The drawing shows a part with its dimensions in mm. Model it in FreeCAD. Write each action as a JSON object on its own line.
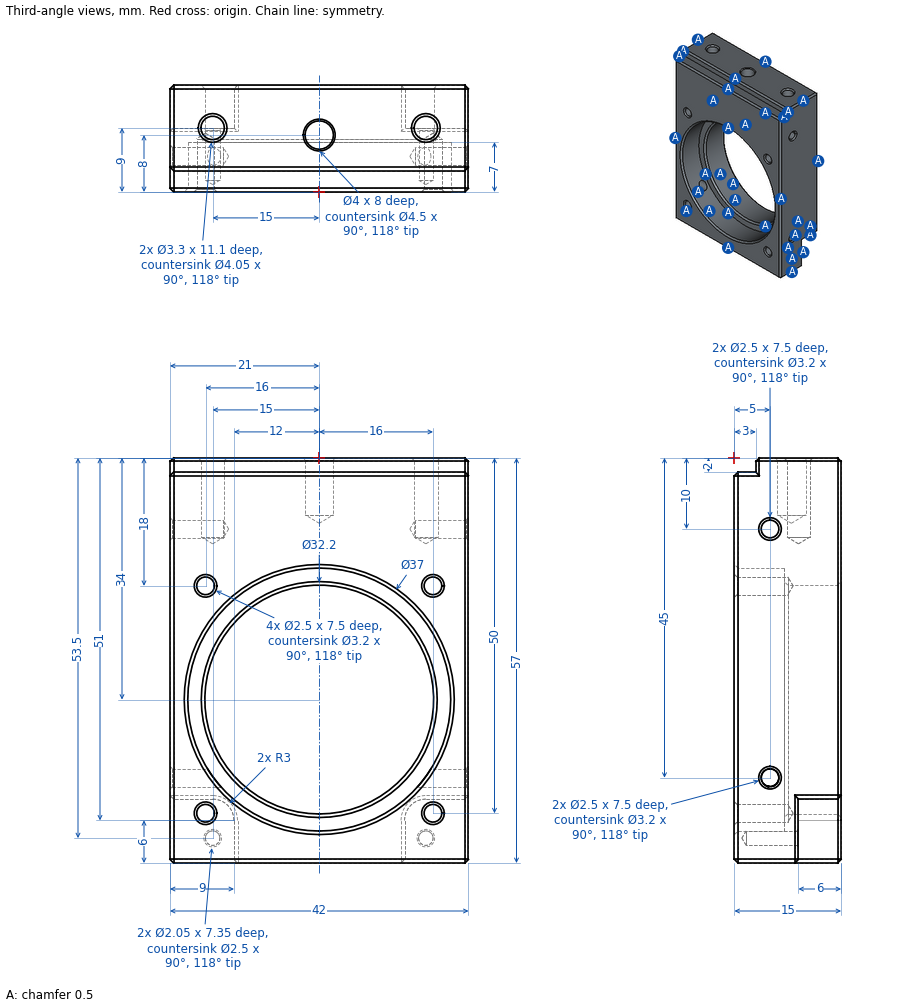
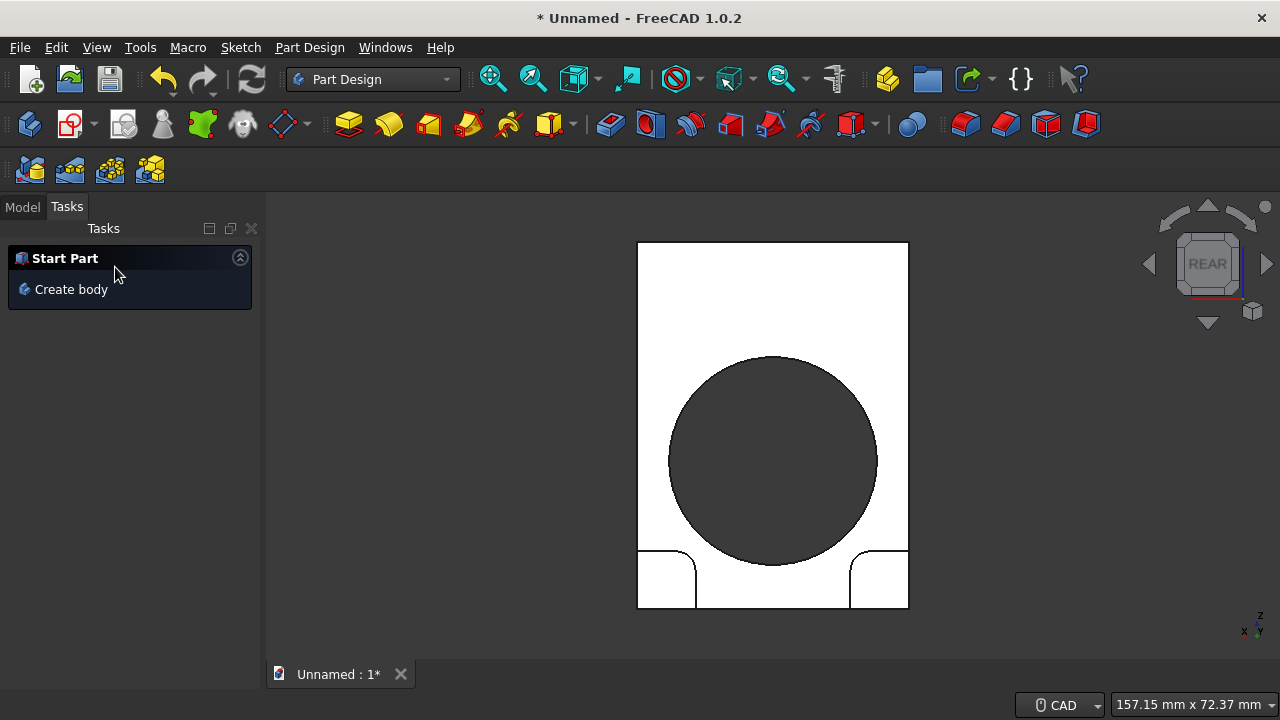
{"action": "left_click", "coordinate": [879, 579]}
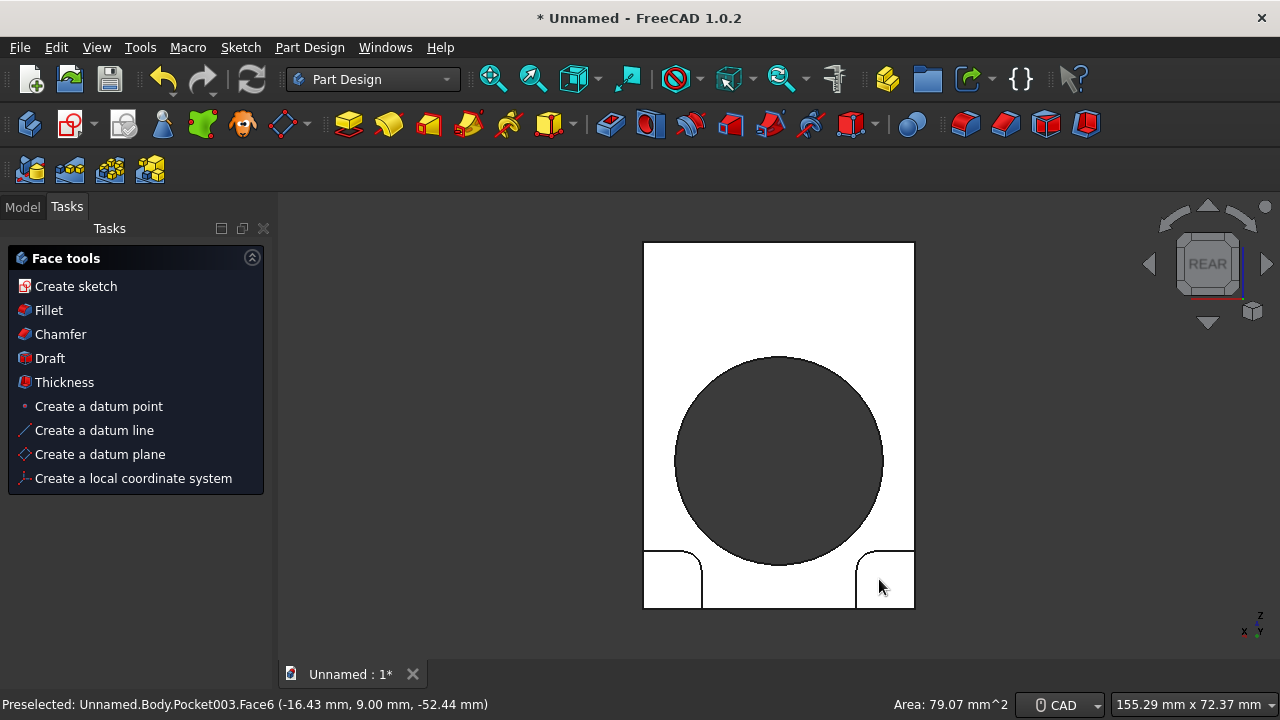
{"action": "left_click", "coordinate": [70, 124]}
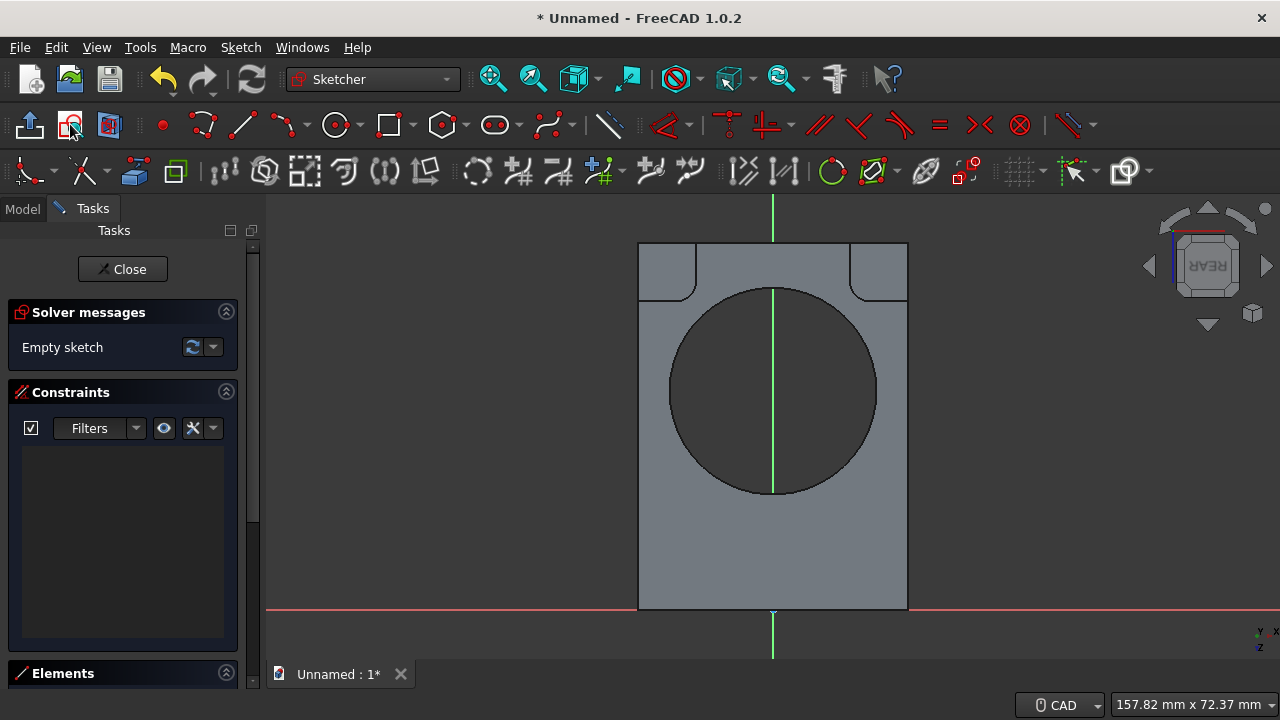
{"action": "key", "text": "q s"}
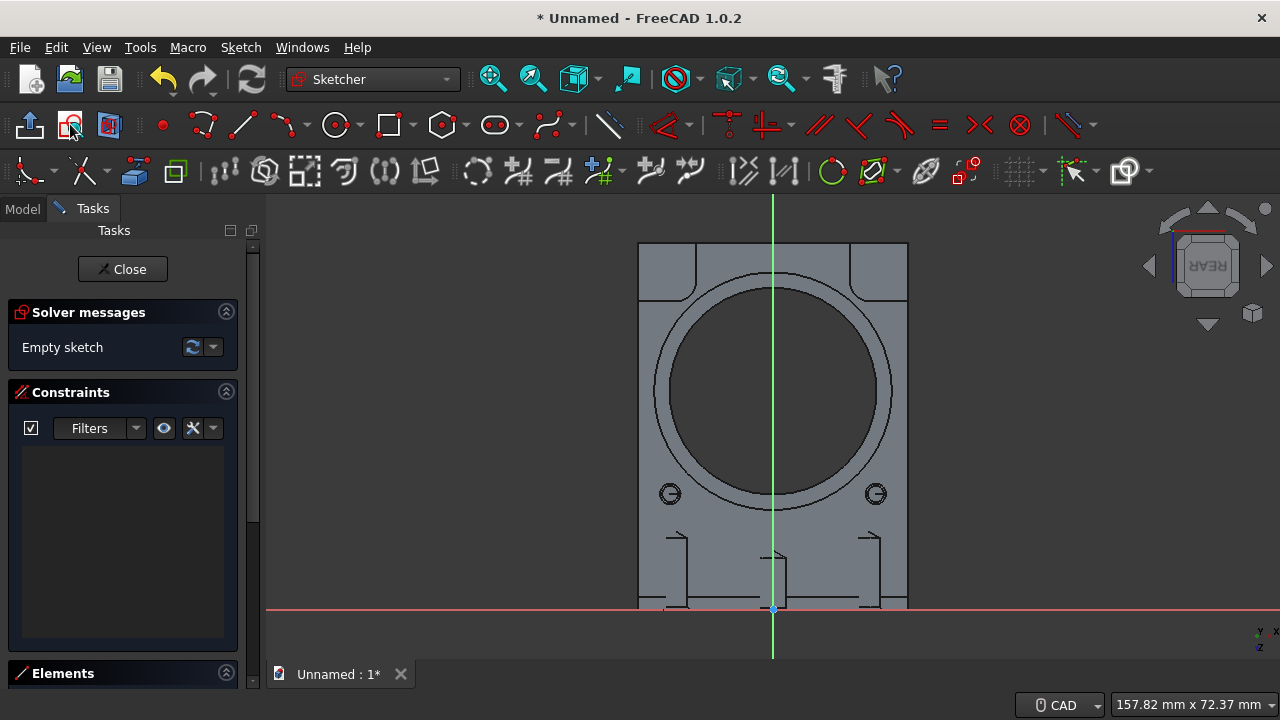
{"action": "scroll", "coordinate": [395, 391], "scroll_direction": "down", "scroll_amount": 1}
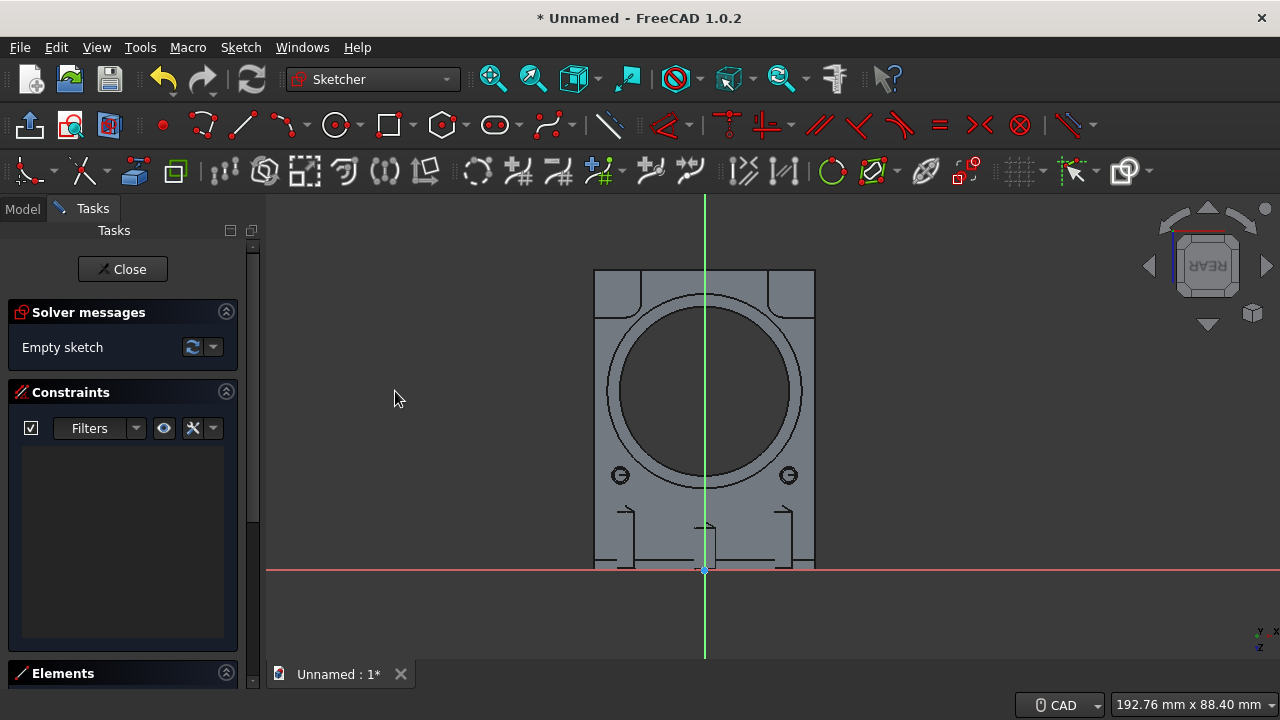
{"action": "key", "text": "g c"}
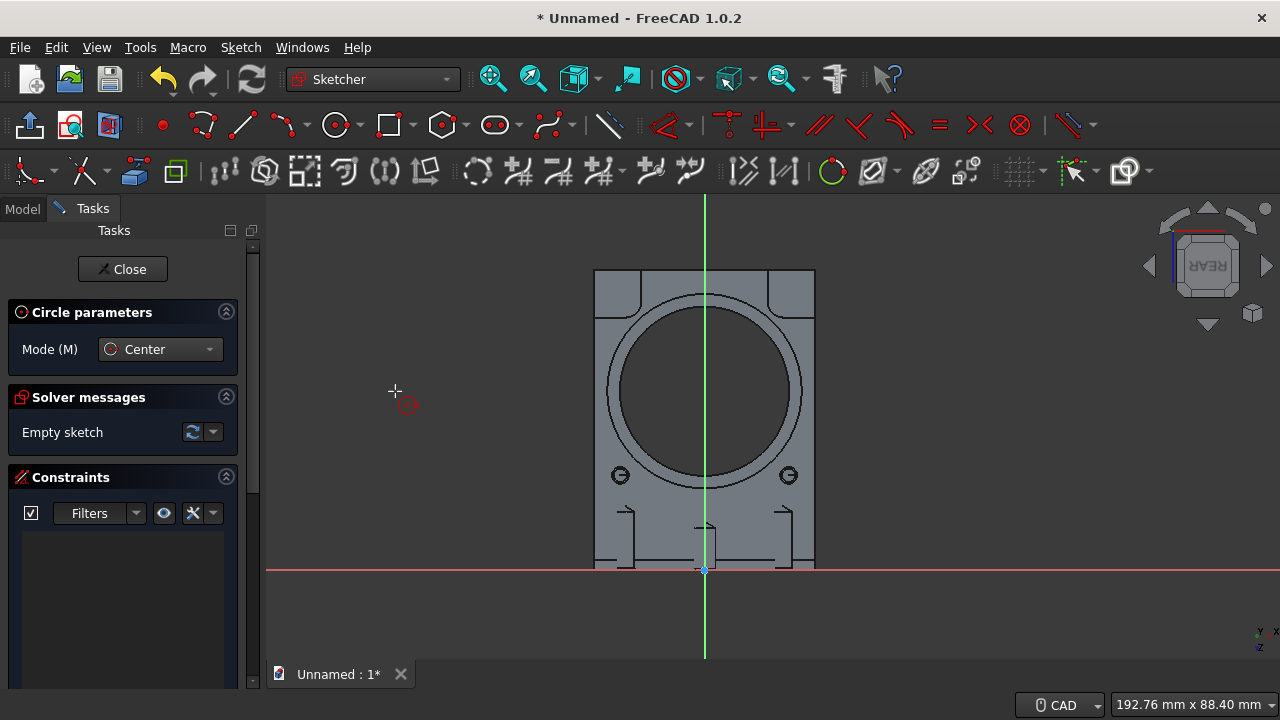
{"action": "scroll", "coordinate": [626, 289], "scroll_direction": "up", "scroll_amount": 8}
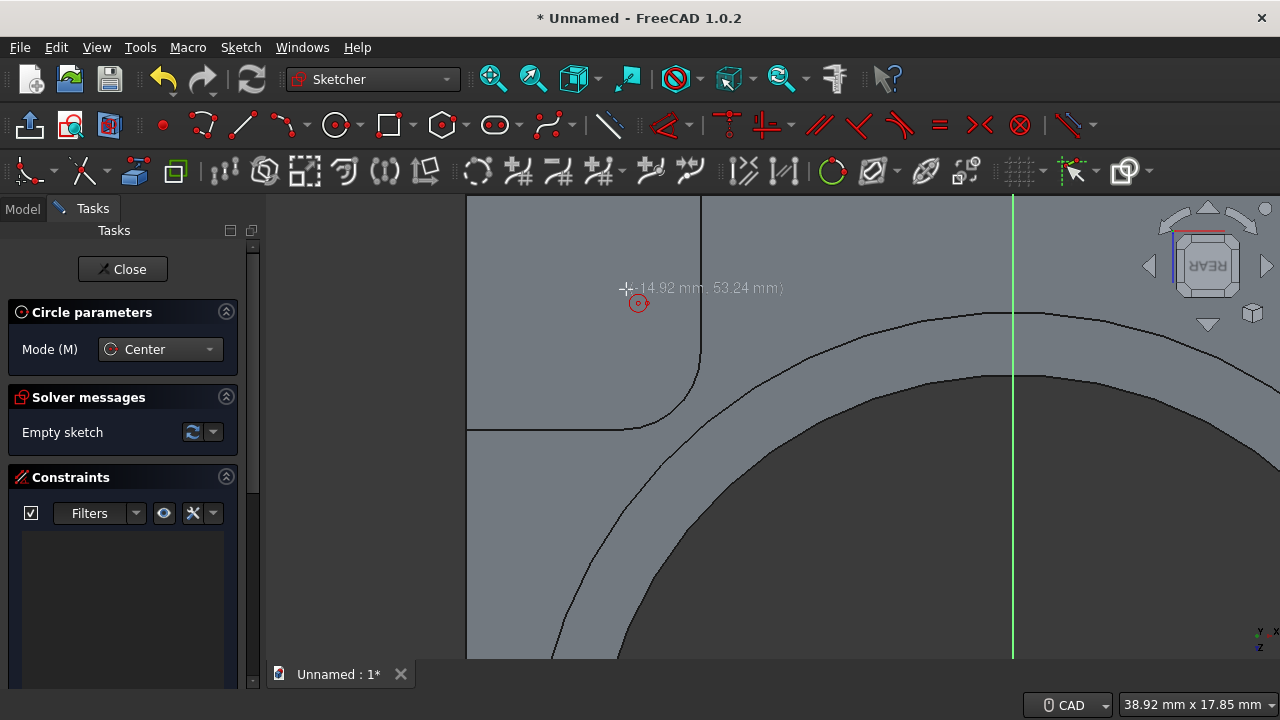
{"action": "scroll", "coordinate": [626, 289], "scroll_direction": "down", "scroll_amount": 8}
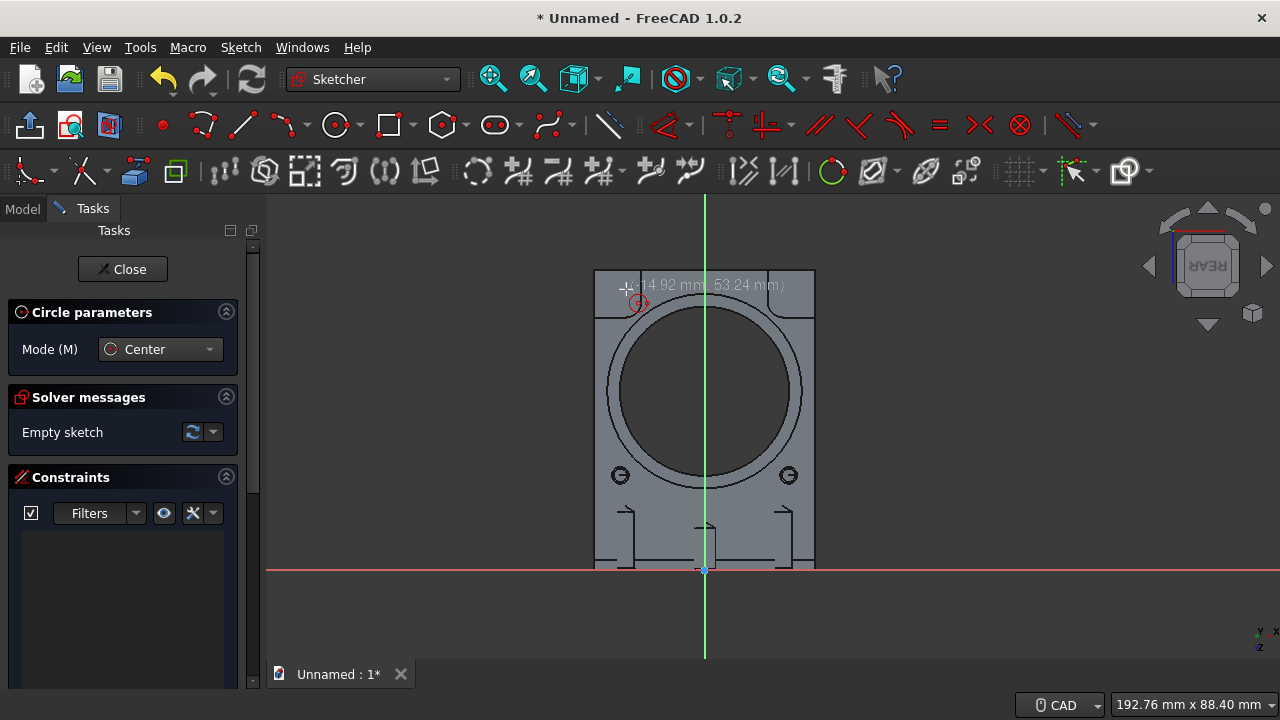
{"action": "left_click", "coordinate": [626, 289]}
{"action": "mouse_move", "coordinate": [629, 285]}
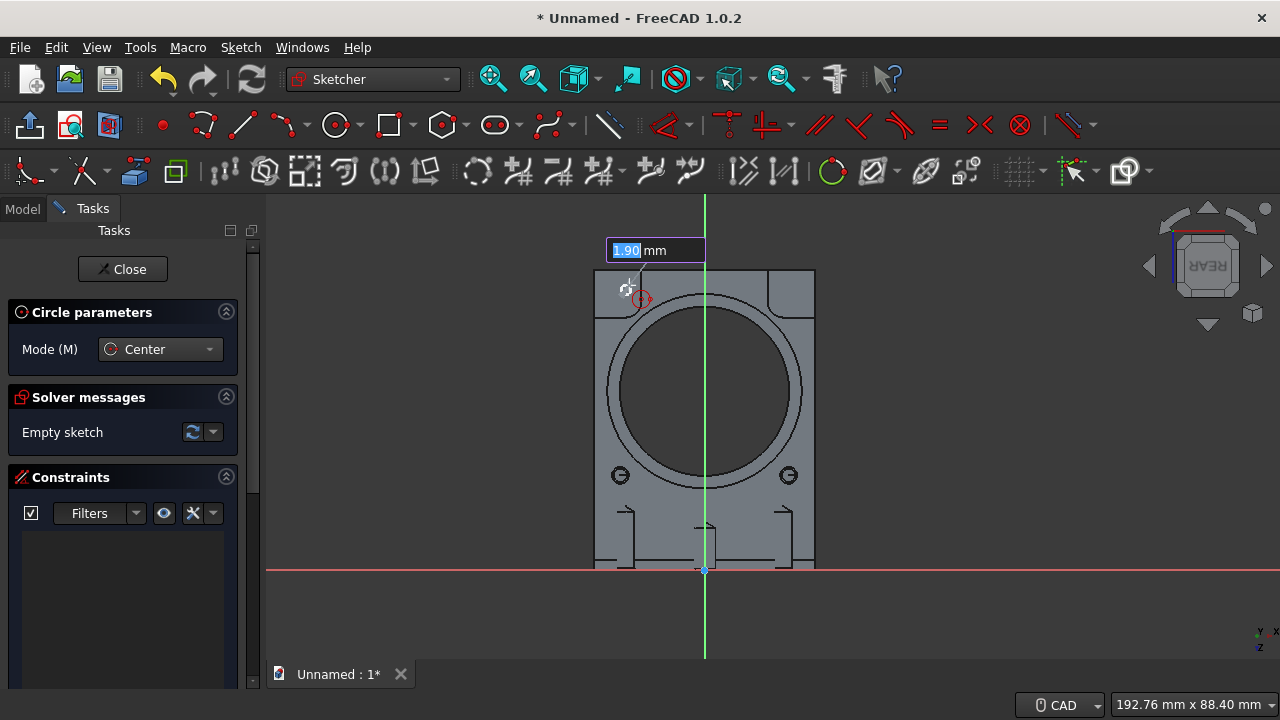
{"action": "type", "text": "2.05"}
{"action": "key", "text": "Return"}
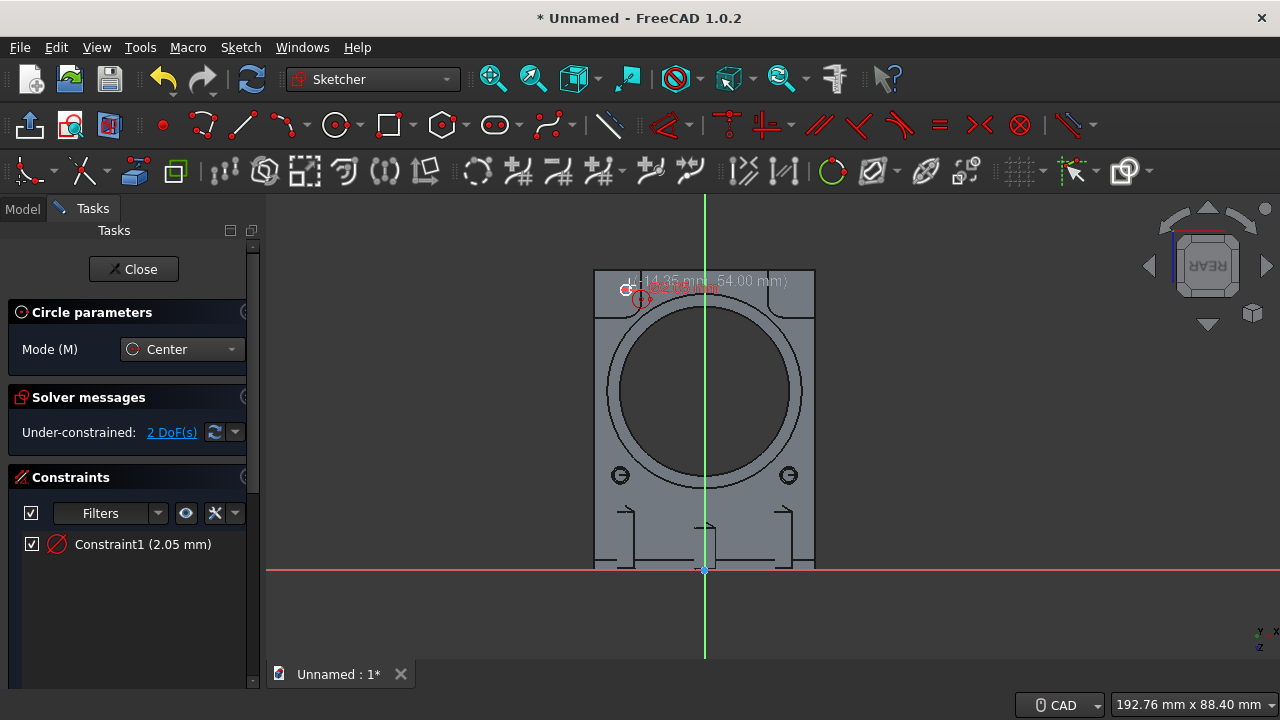
{"action": "scroll", "coordinate": [783, 289], "scroll_direction": "up", "scroll_amount": 8}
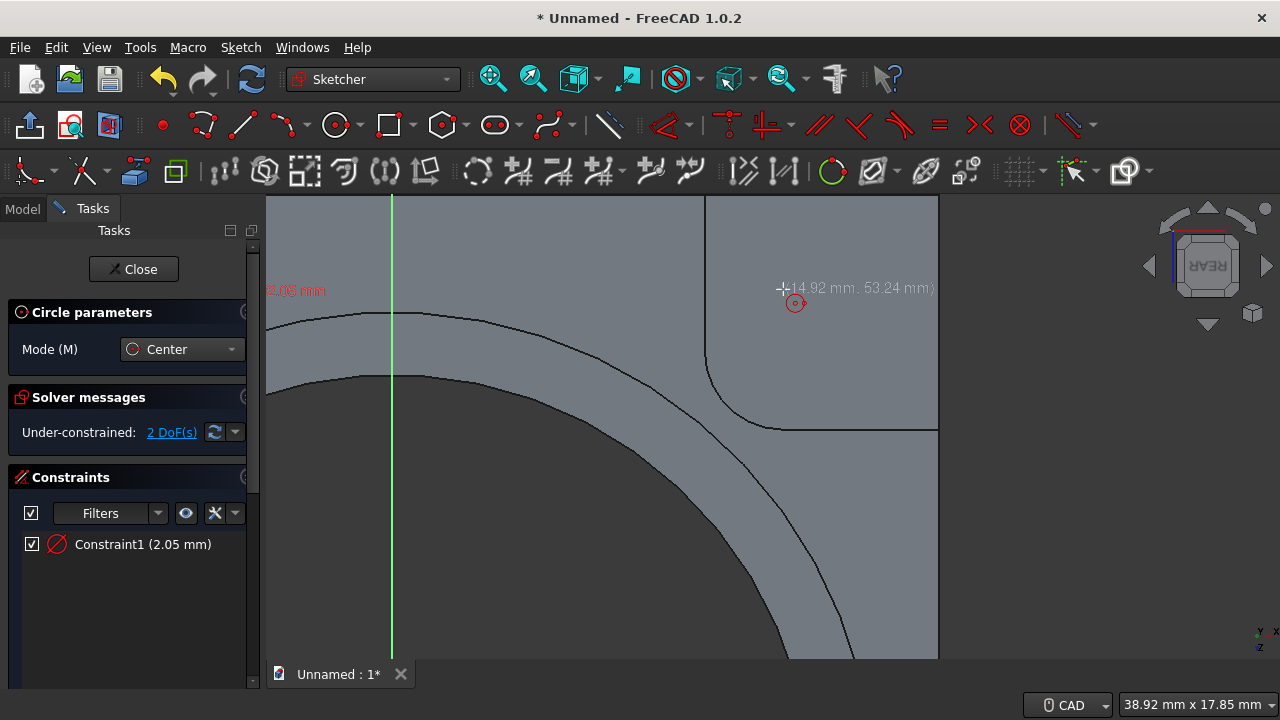
{"action": "scroll", "coordinate": [784, 289], "scroll_direction": "down", "scroll_amount": 8}